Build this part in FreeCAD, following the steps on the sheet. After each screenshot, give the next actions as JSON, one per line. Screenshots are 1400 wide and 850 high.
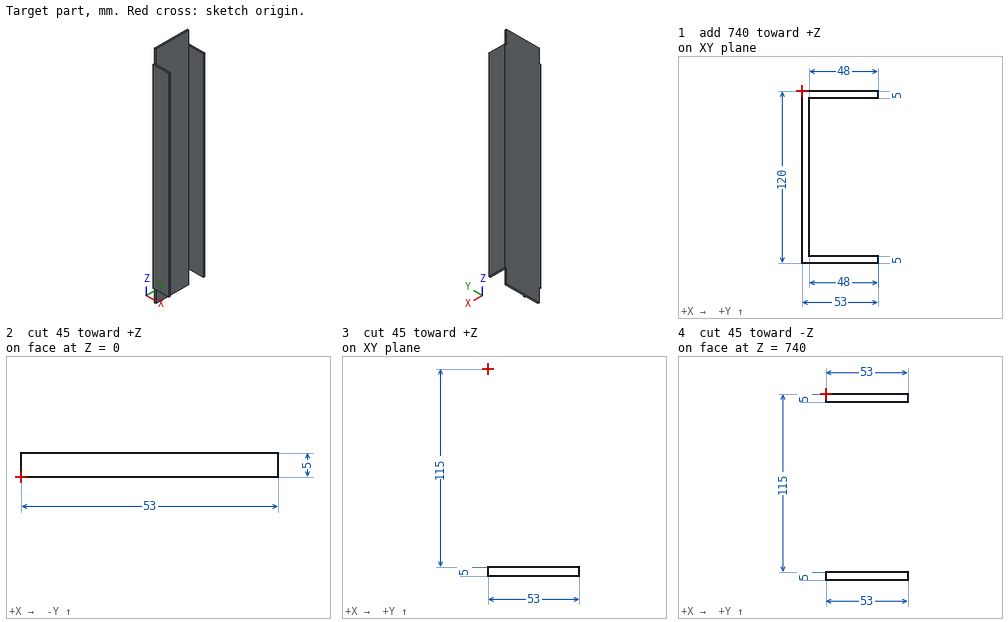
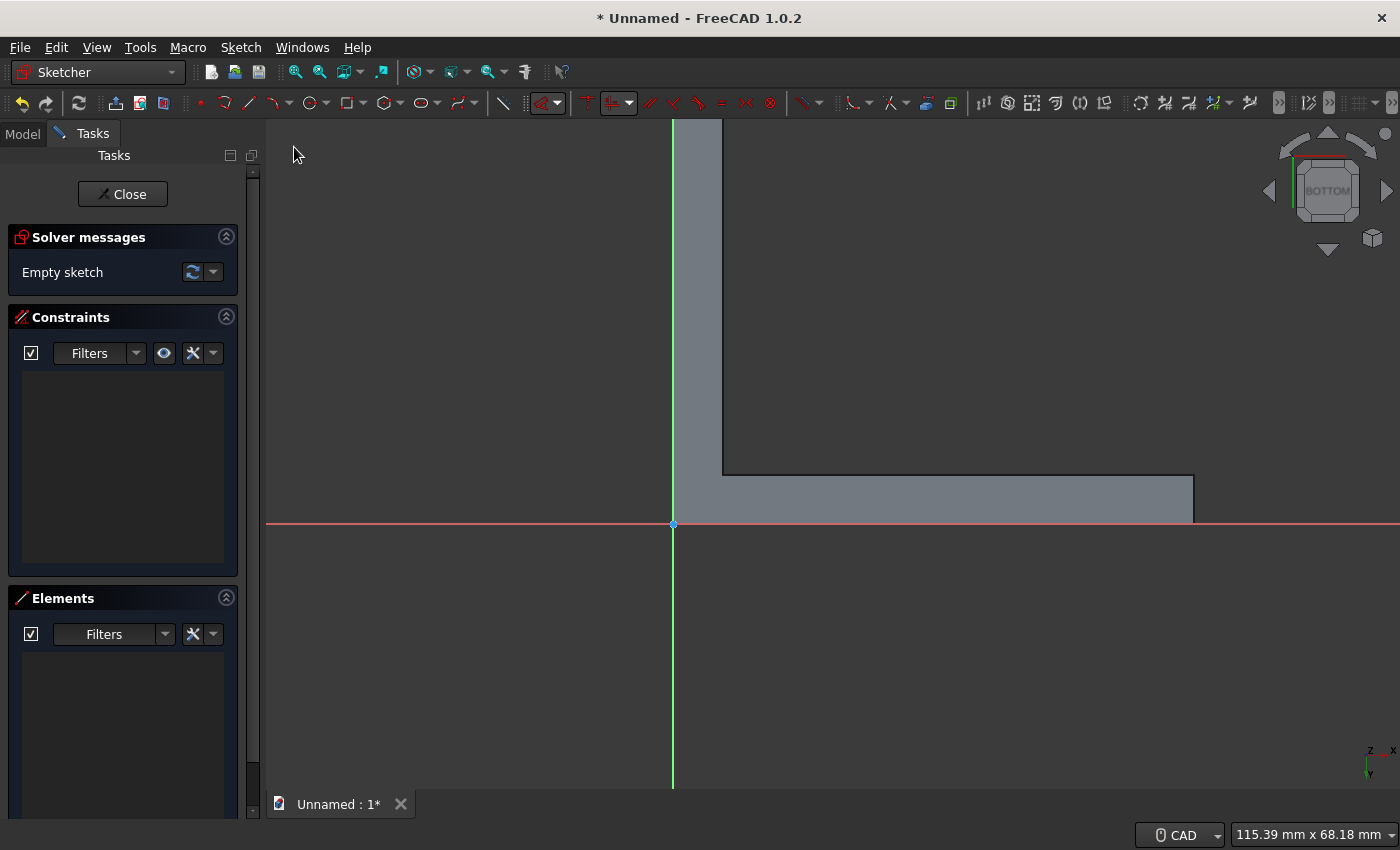
{"action": "left_click", "coordinate": [348, 104]}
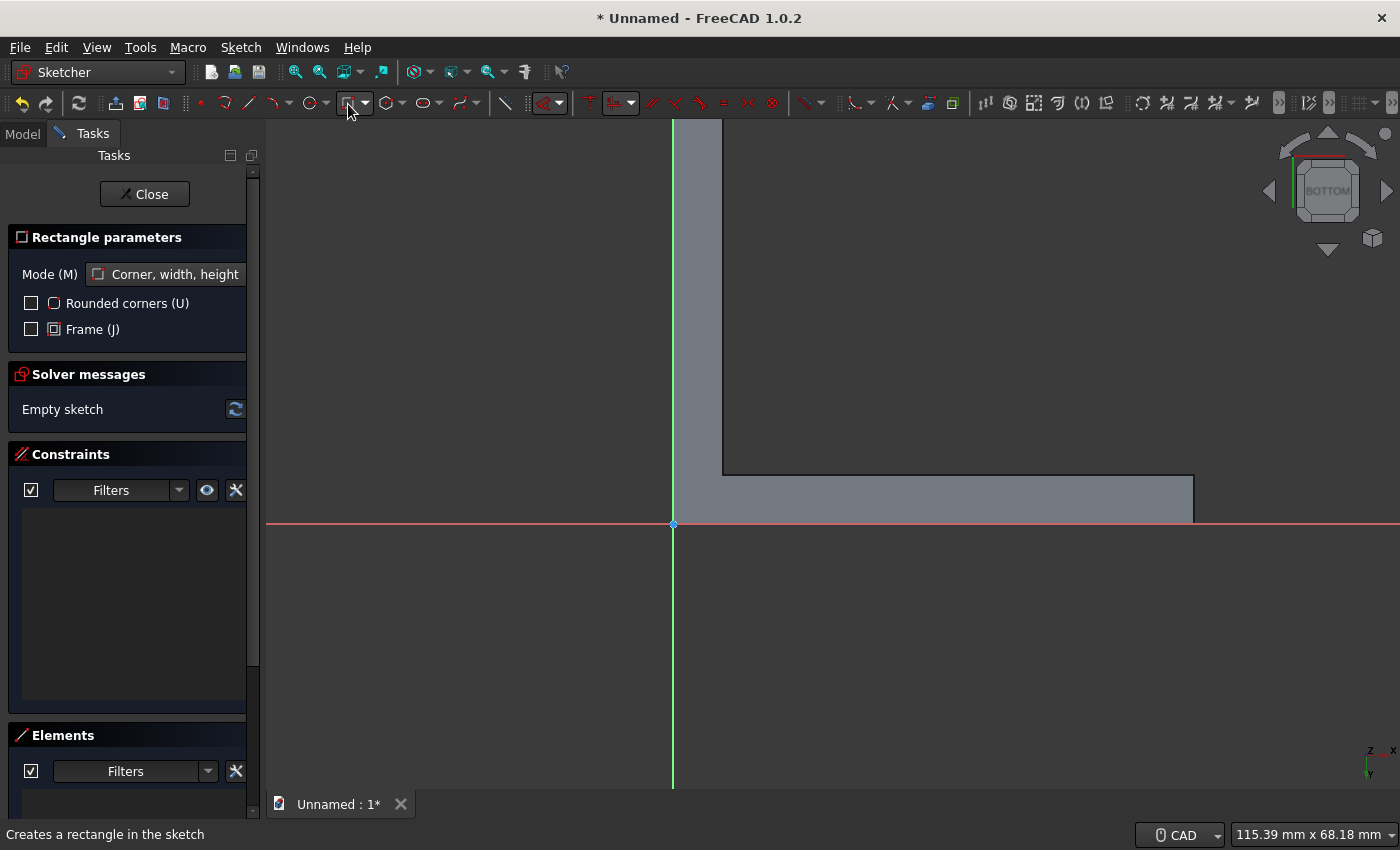
{"action": "left_click", "coordinate": [673, 524]}
{"action": "left_click", "coordinate": [1194, 475]}
{"action": "key", "text": "Escape"}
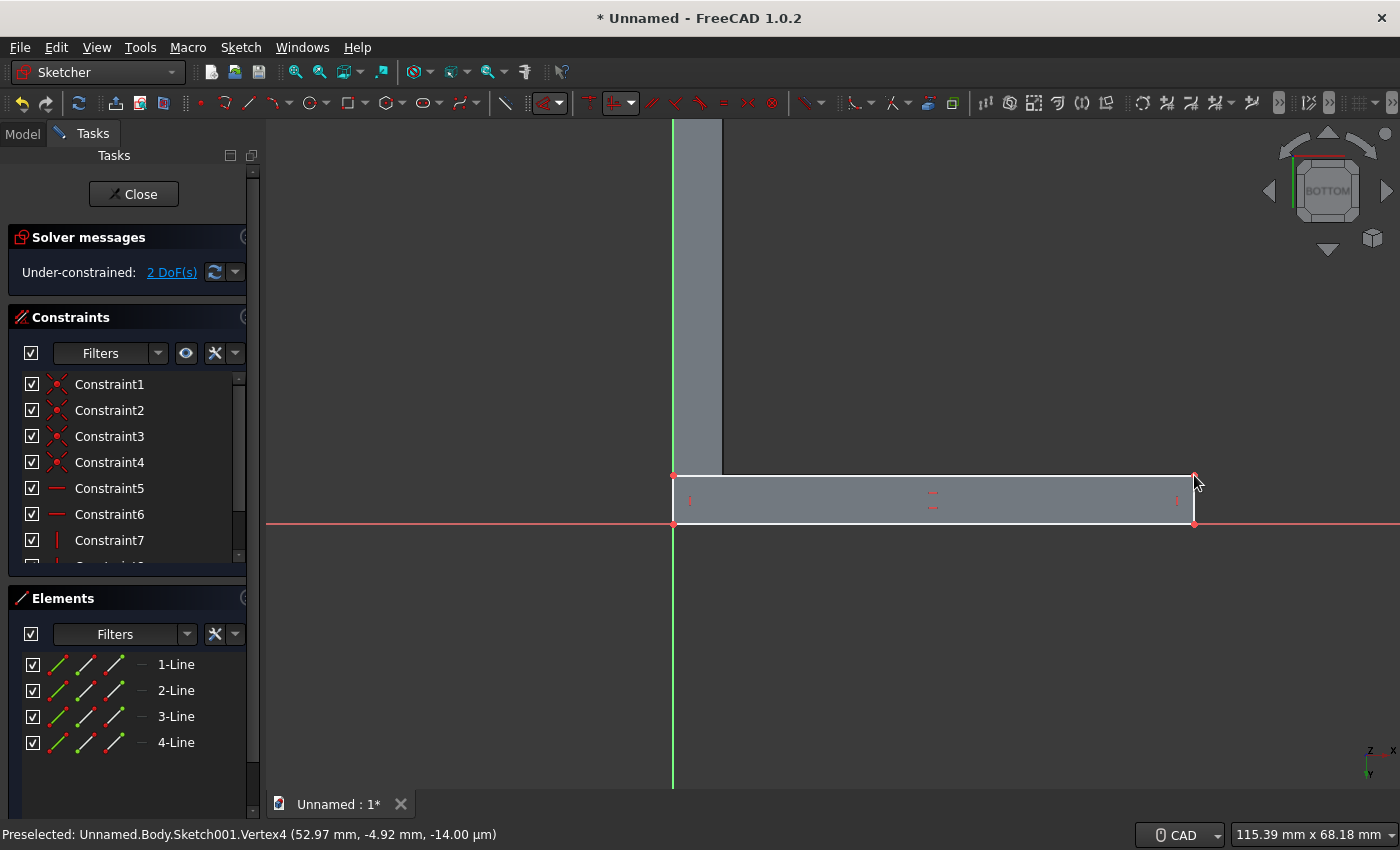
{"action": "left_click", "coordinate": [1194, 510]}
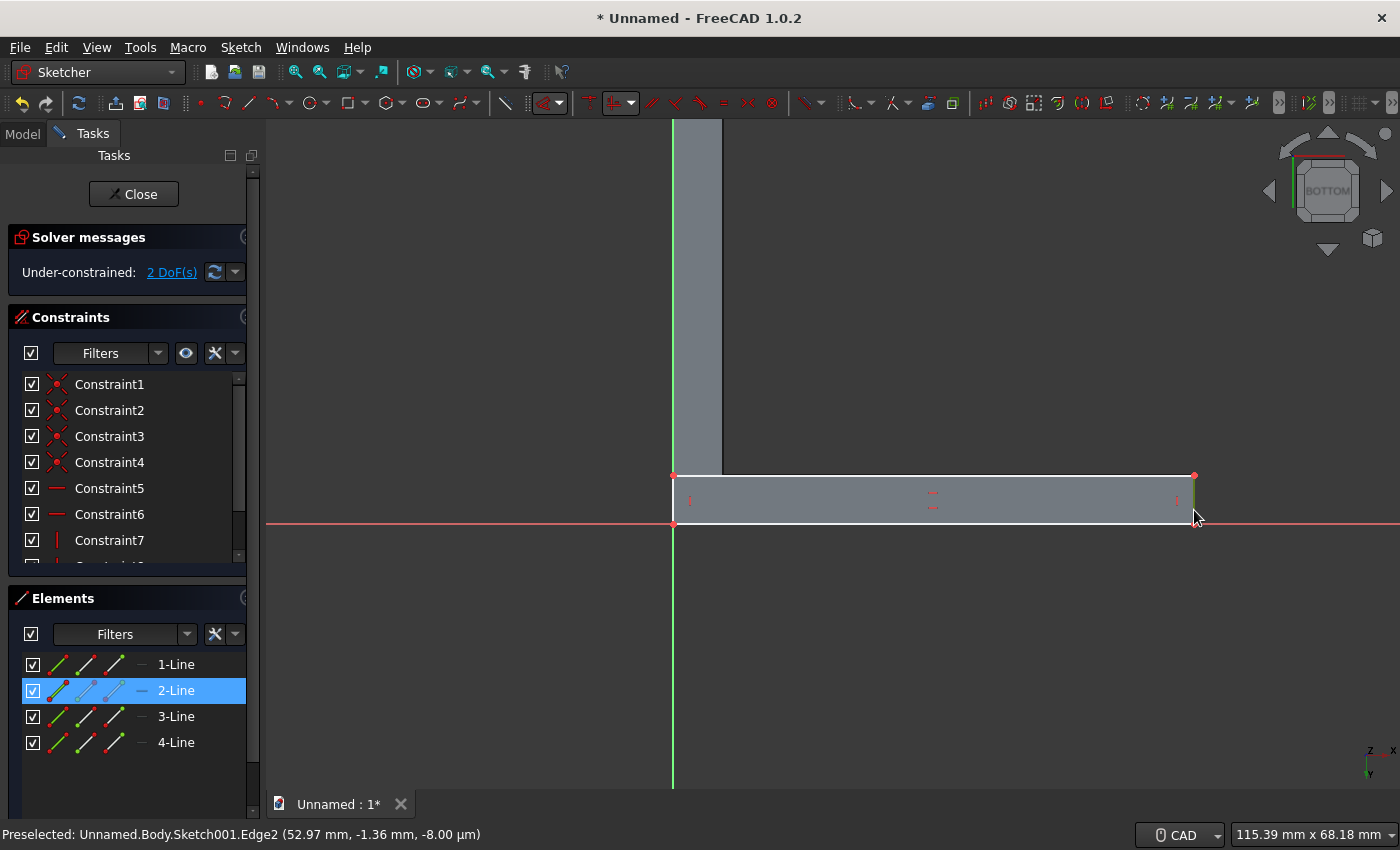
{"action": "key", "text": "i"}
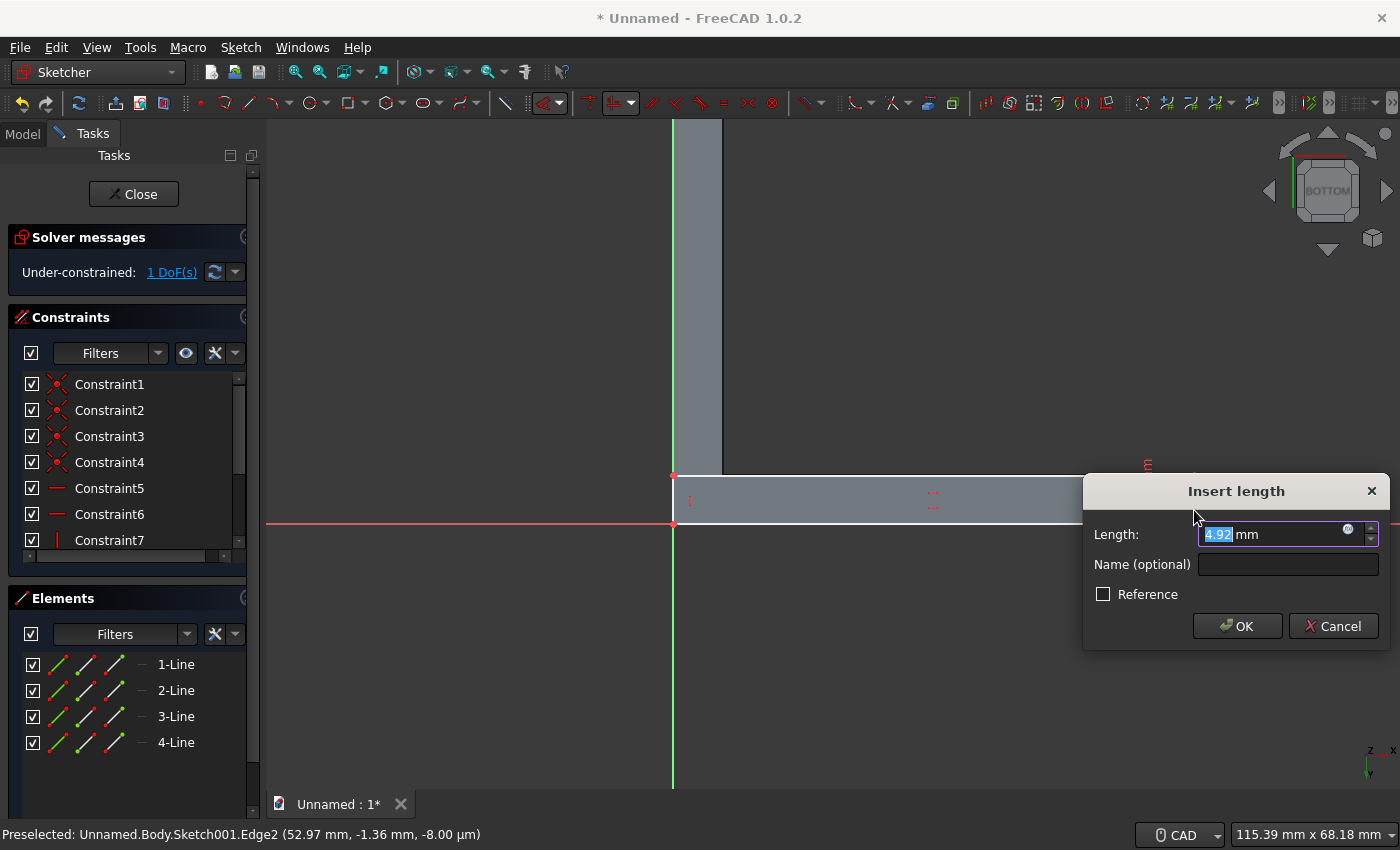
{"action": "type", "text": "5"}
{"action": "key", "text": "Return"}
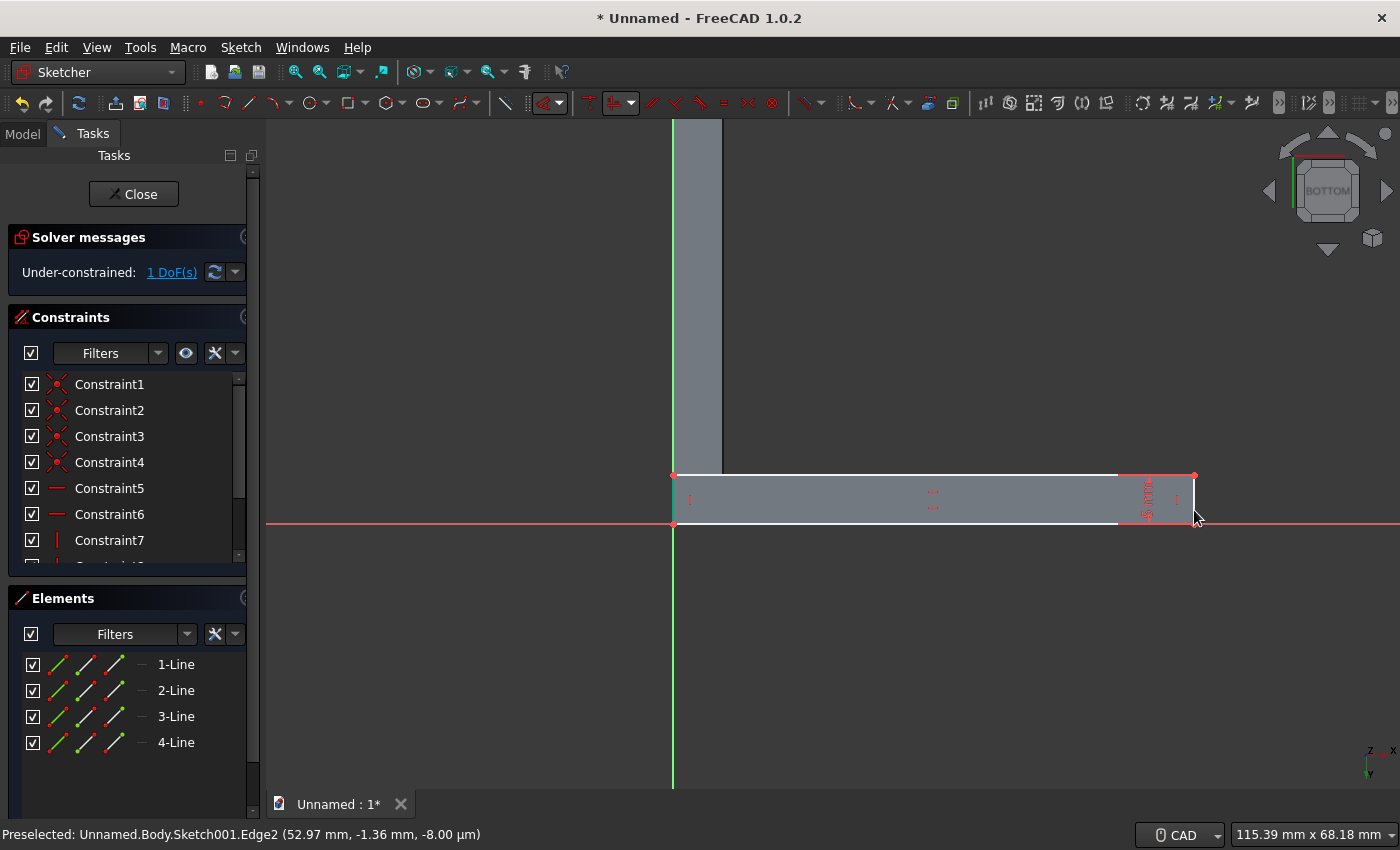
{"action": "left_click", "coordinate": [830, 524]}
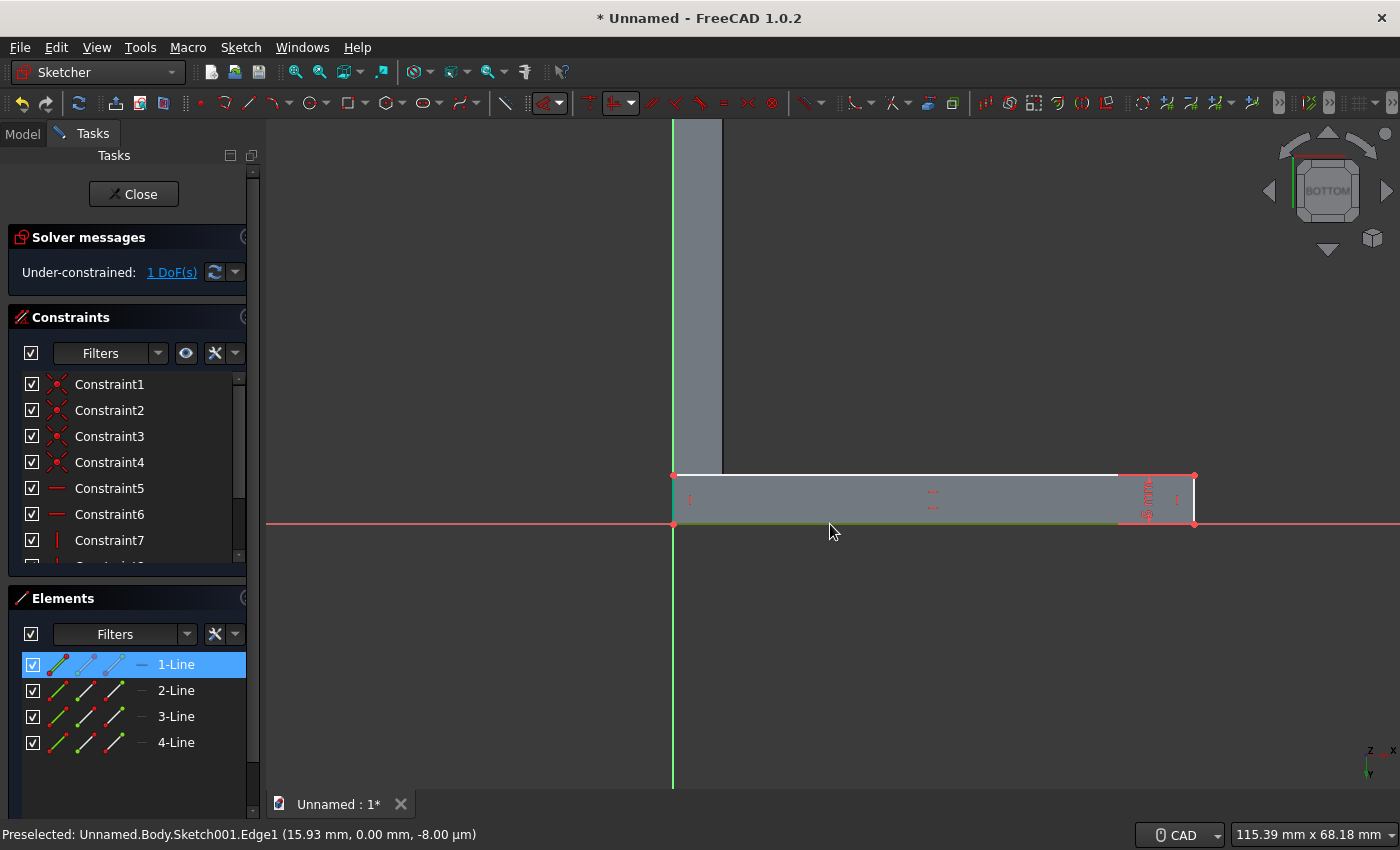
{"action": "key", "text": "l"}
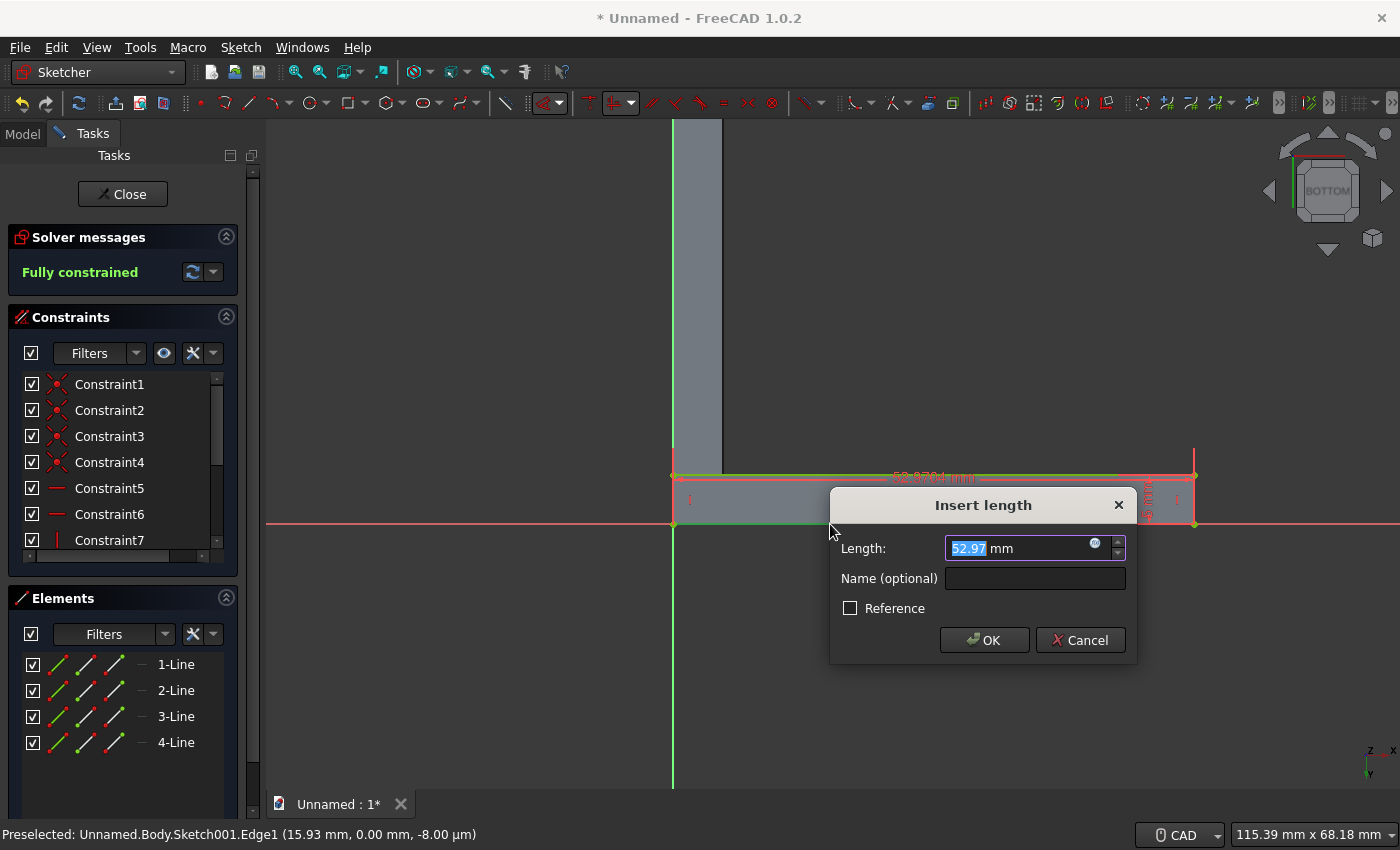
{"action": "type", "text": "53"}
{"action": "key", "text": "Return"}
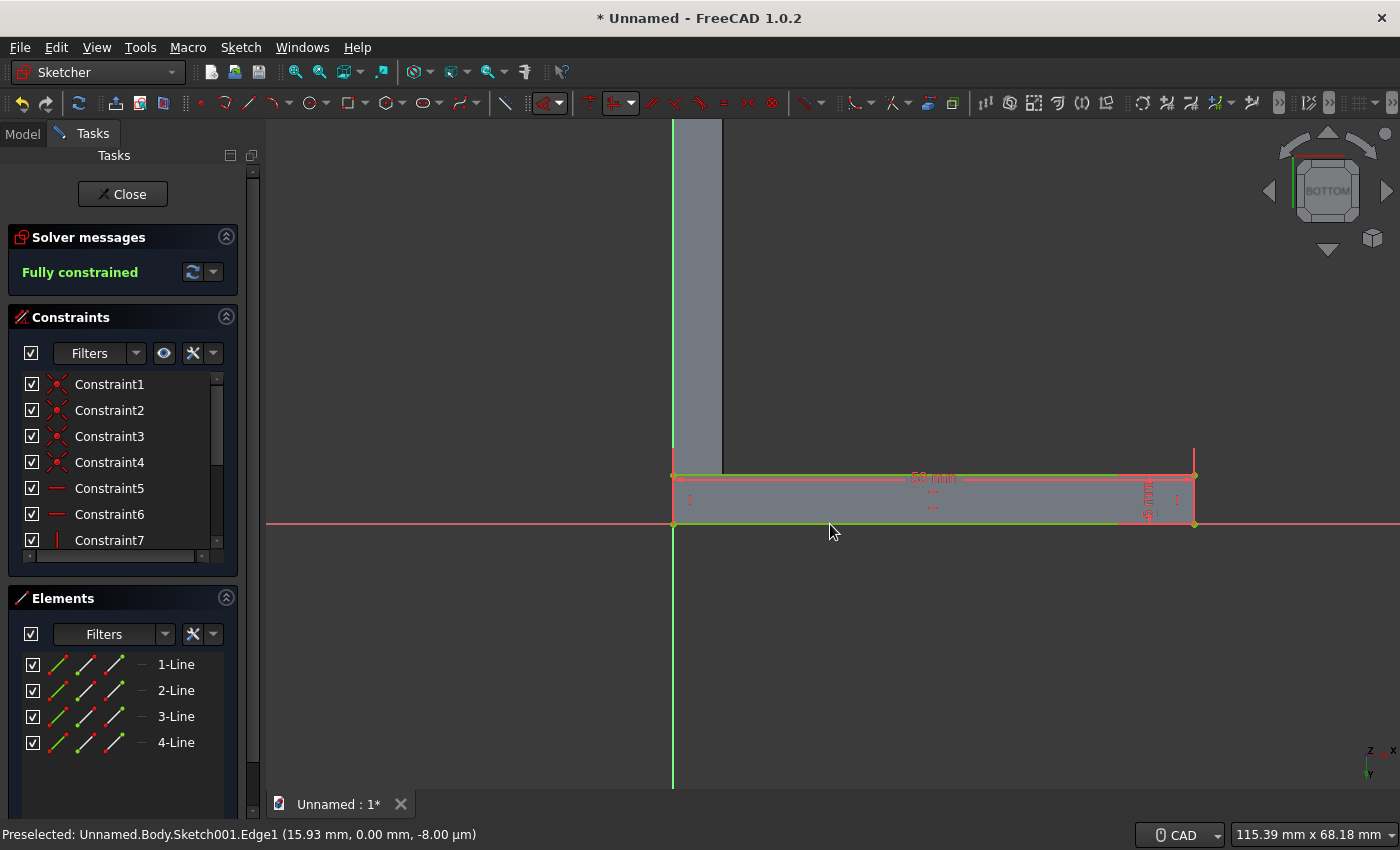
{"action": "left_click", "coordinate": [123, 194]}